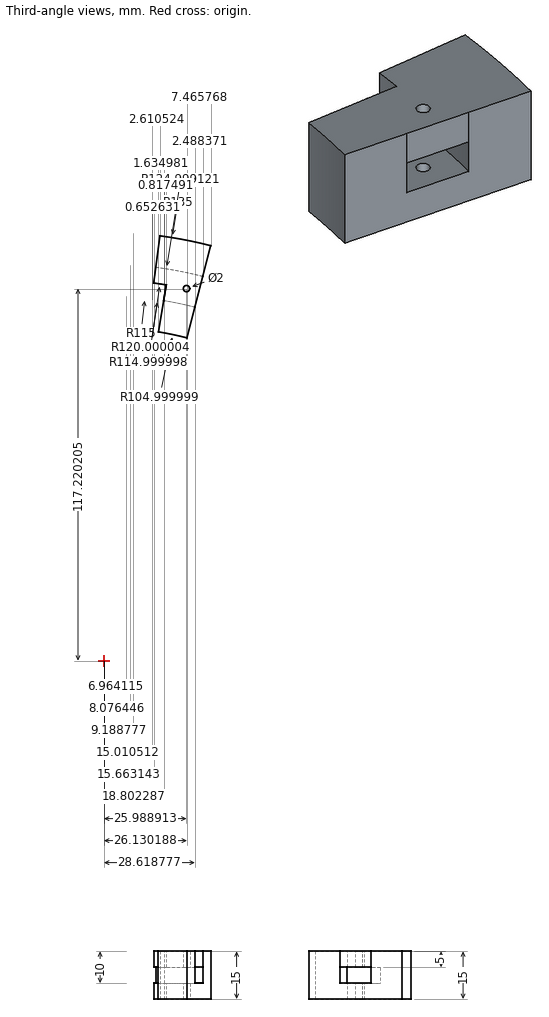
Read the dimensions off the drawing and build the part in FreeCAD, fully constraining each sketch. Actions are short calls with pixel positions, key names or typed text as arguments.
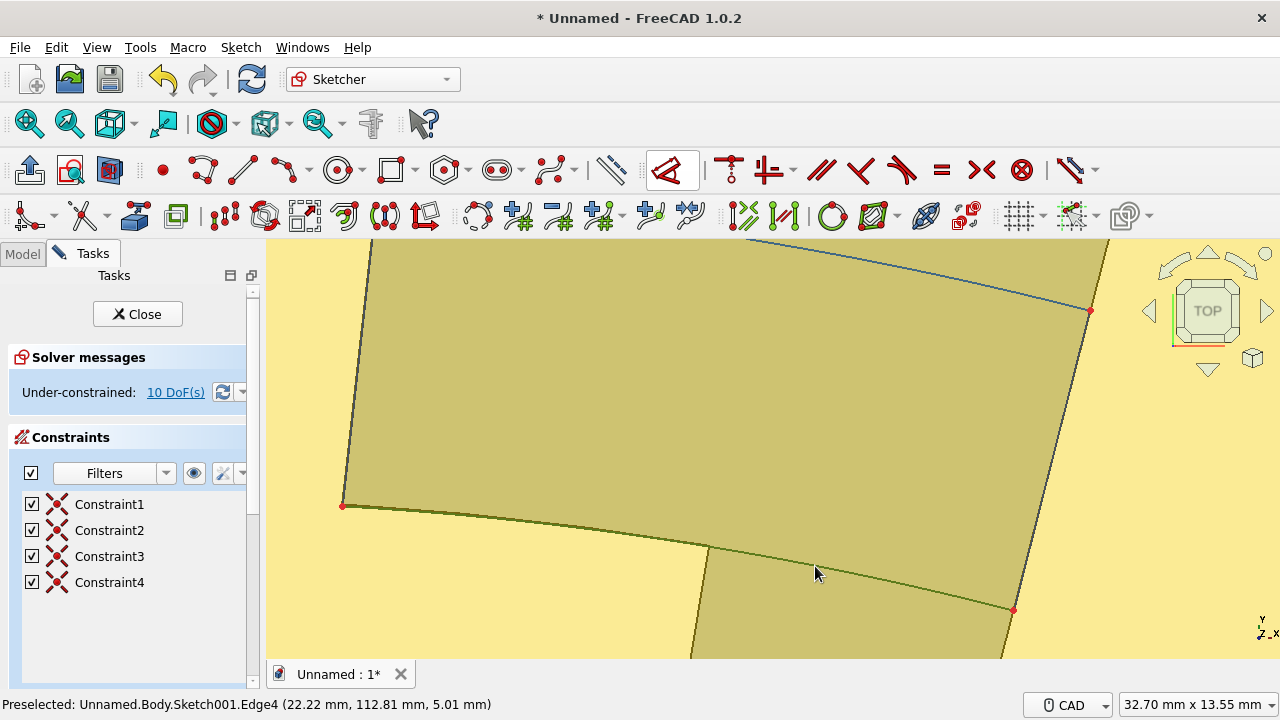
click(730, 170)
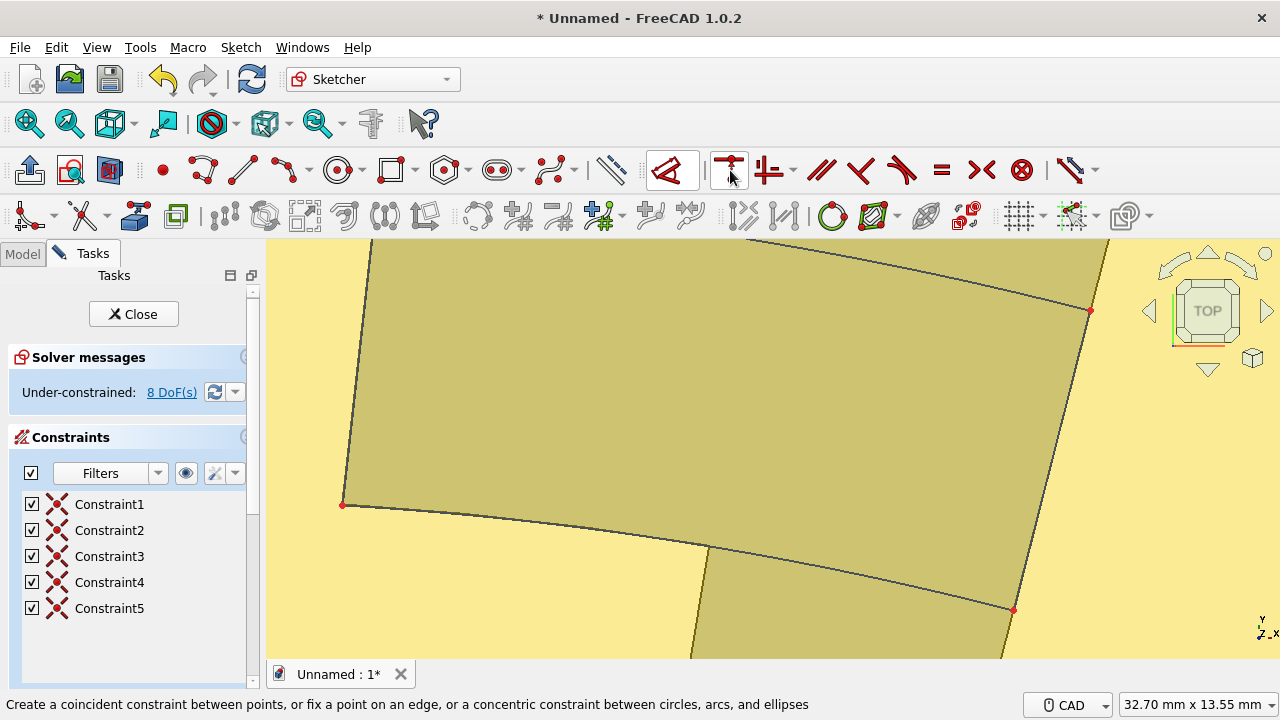
scroll(680, 543, down, 2)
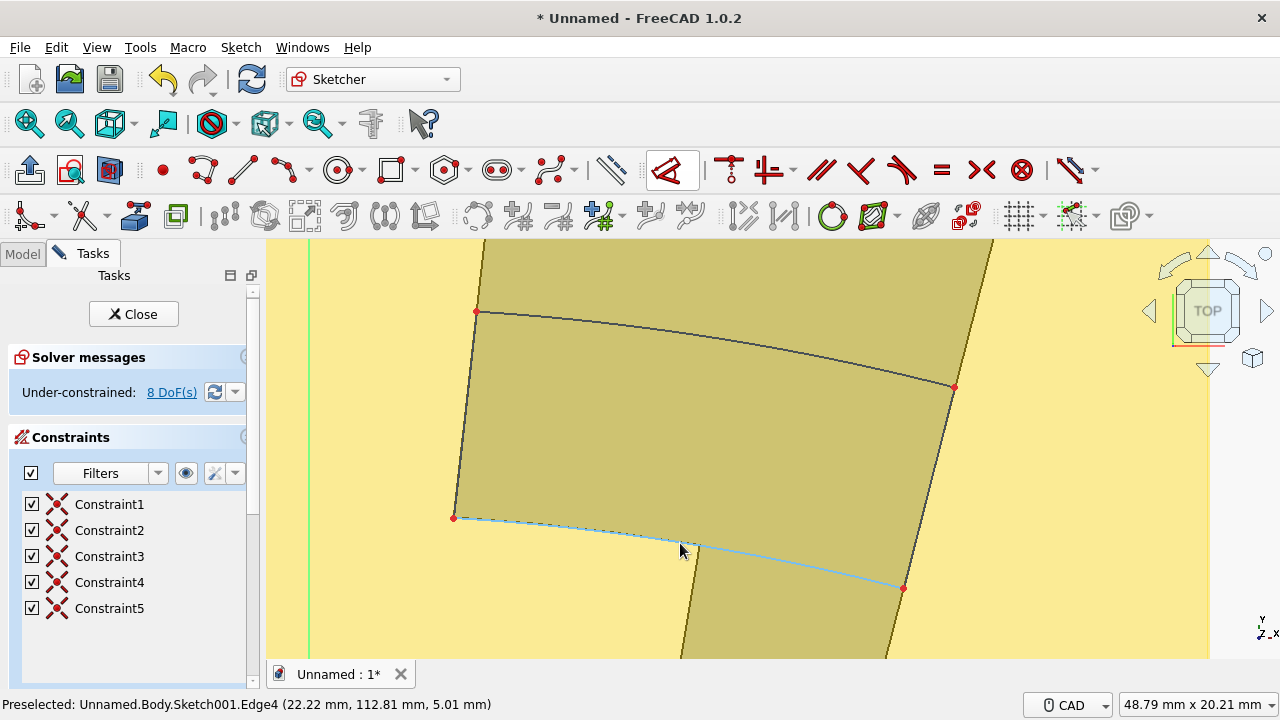
scroll(712, 334, down, 12)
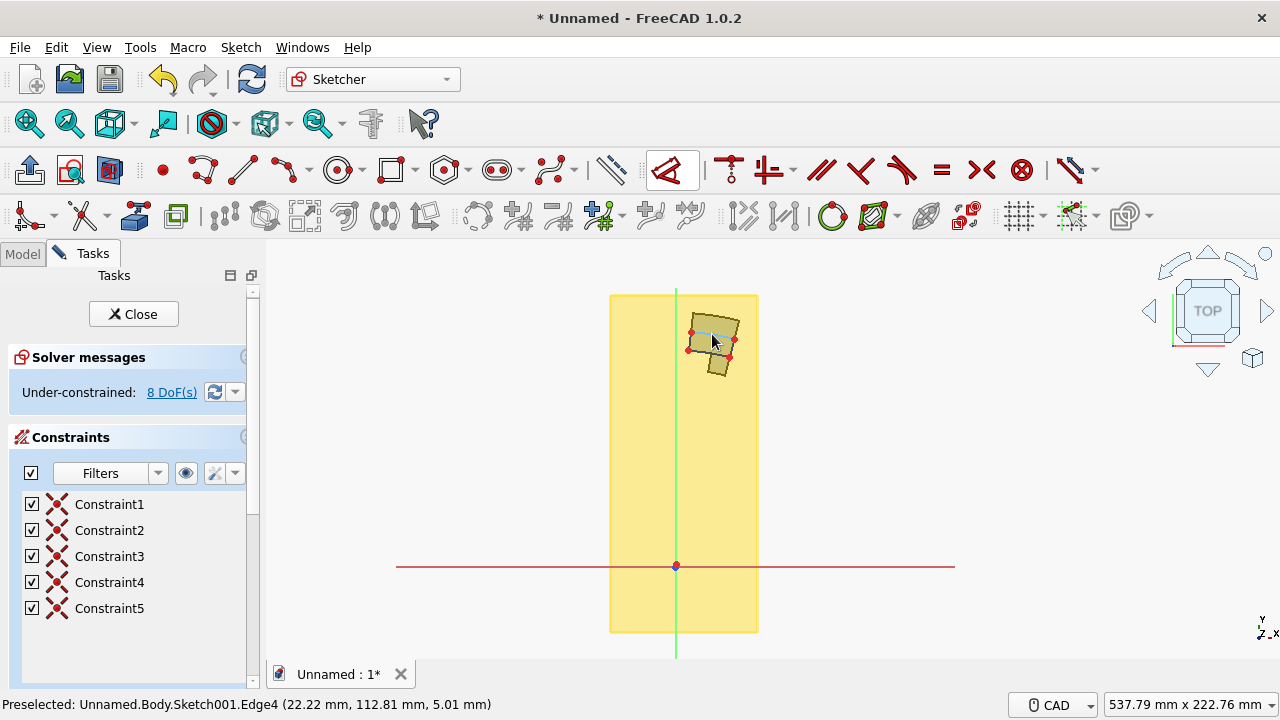
drag(666, 554, 686, 577)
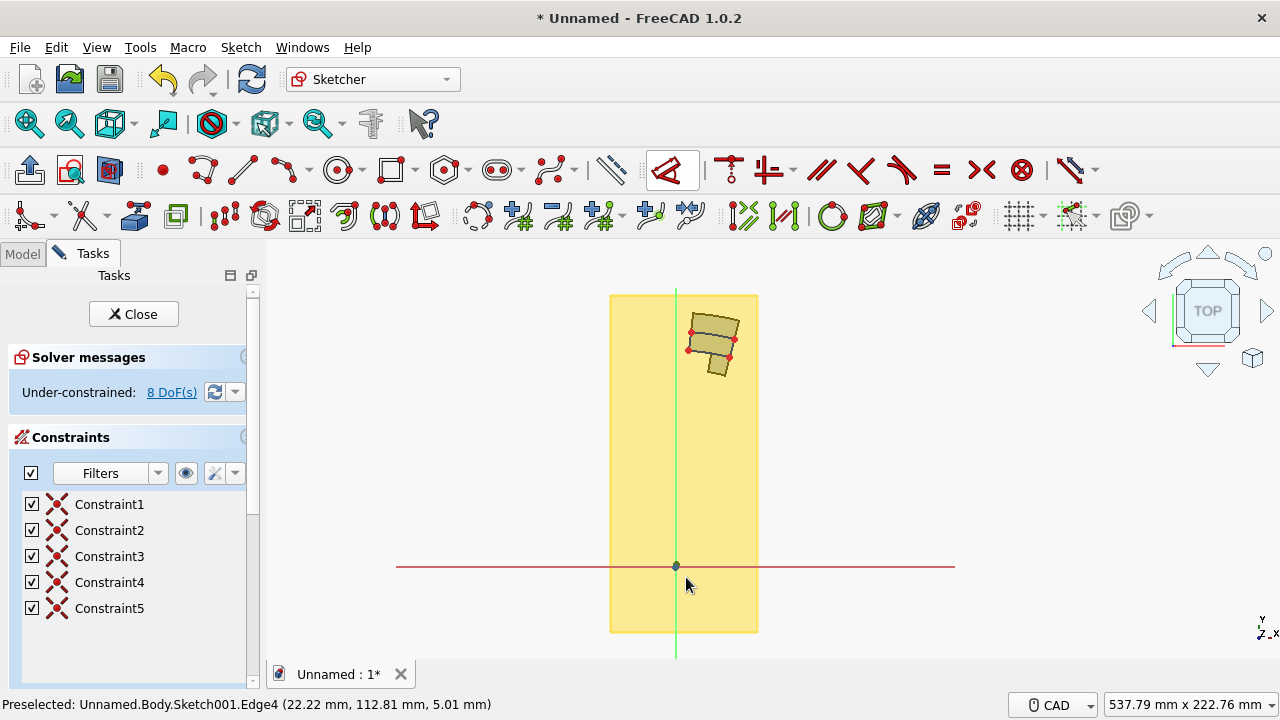
click(730, 170)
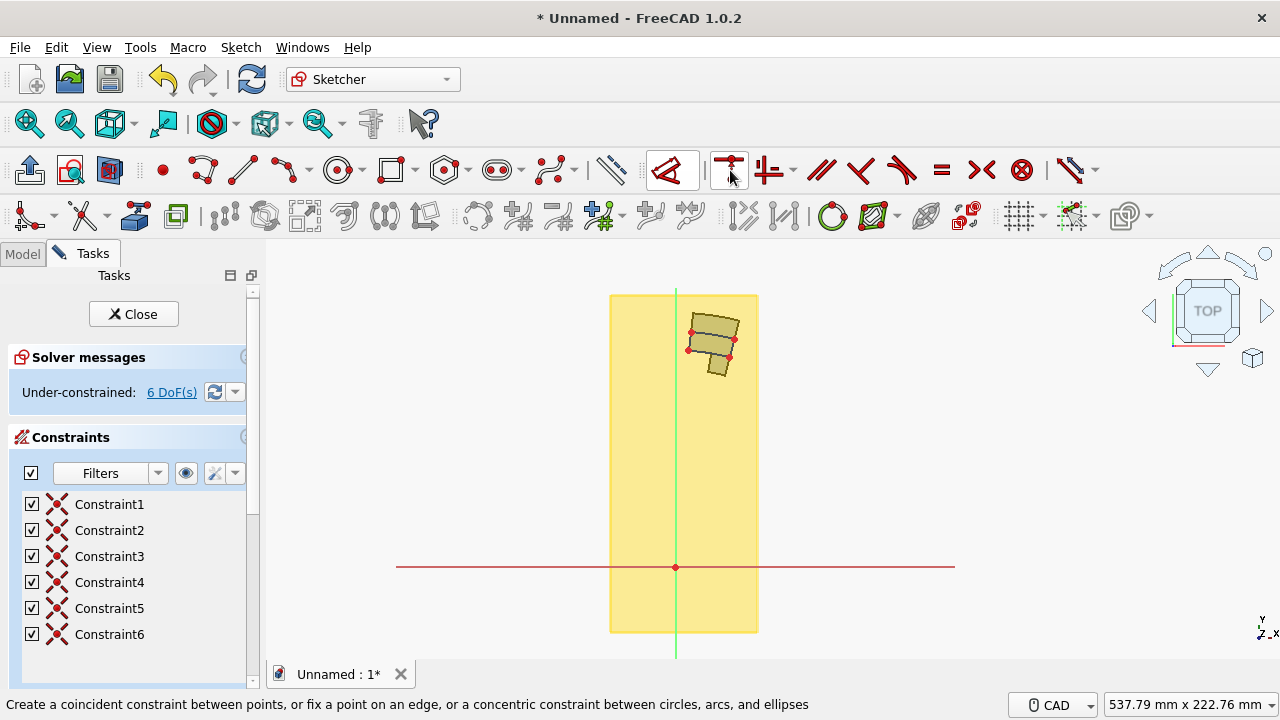
click(722, 336)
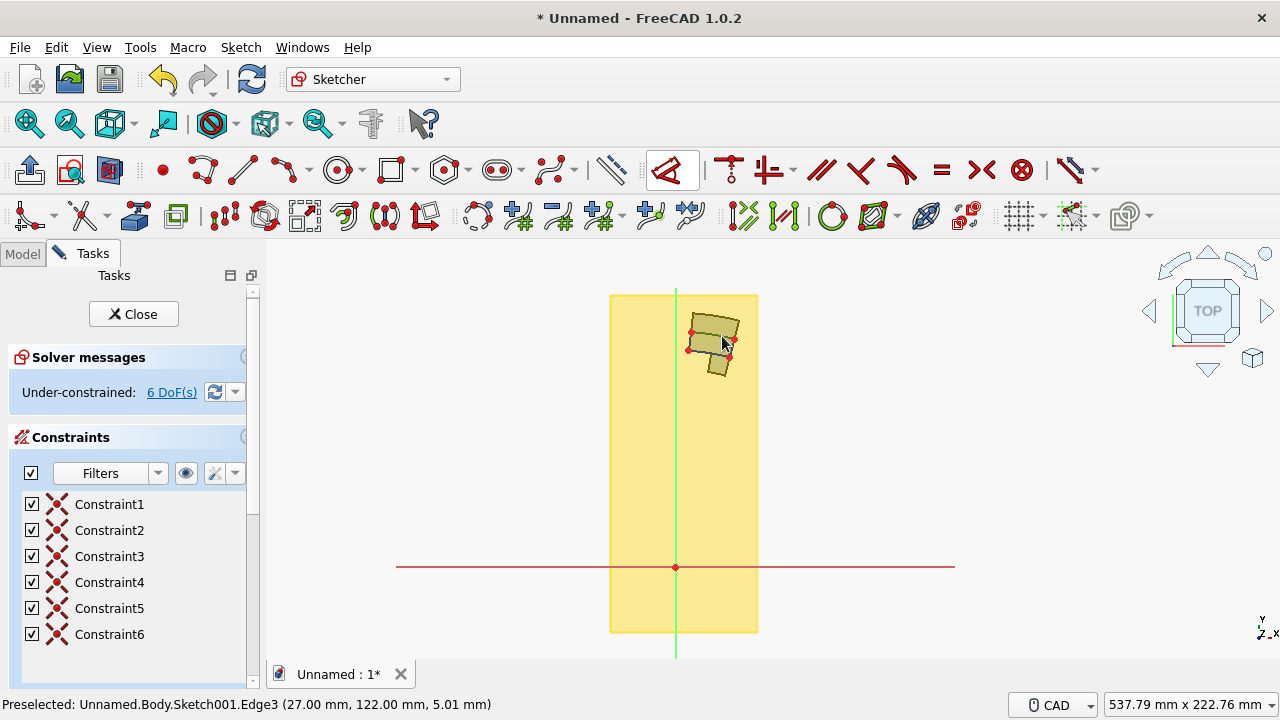
key(k)
key(r)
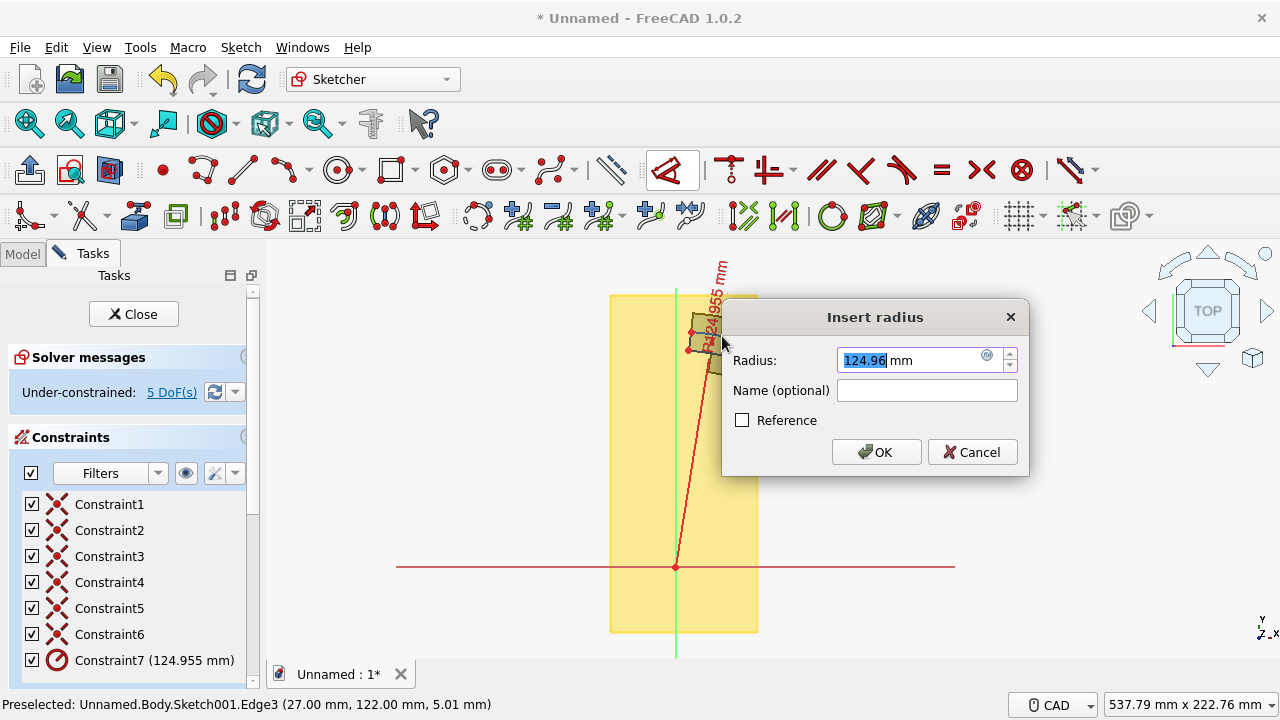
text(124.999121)
key(Return)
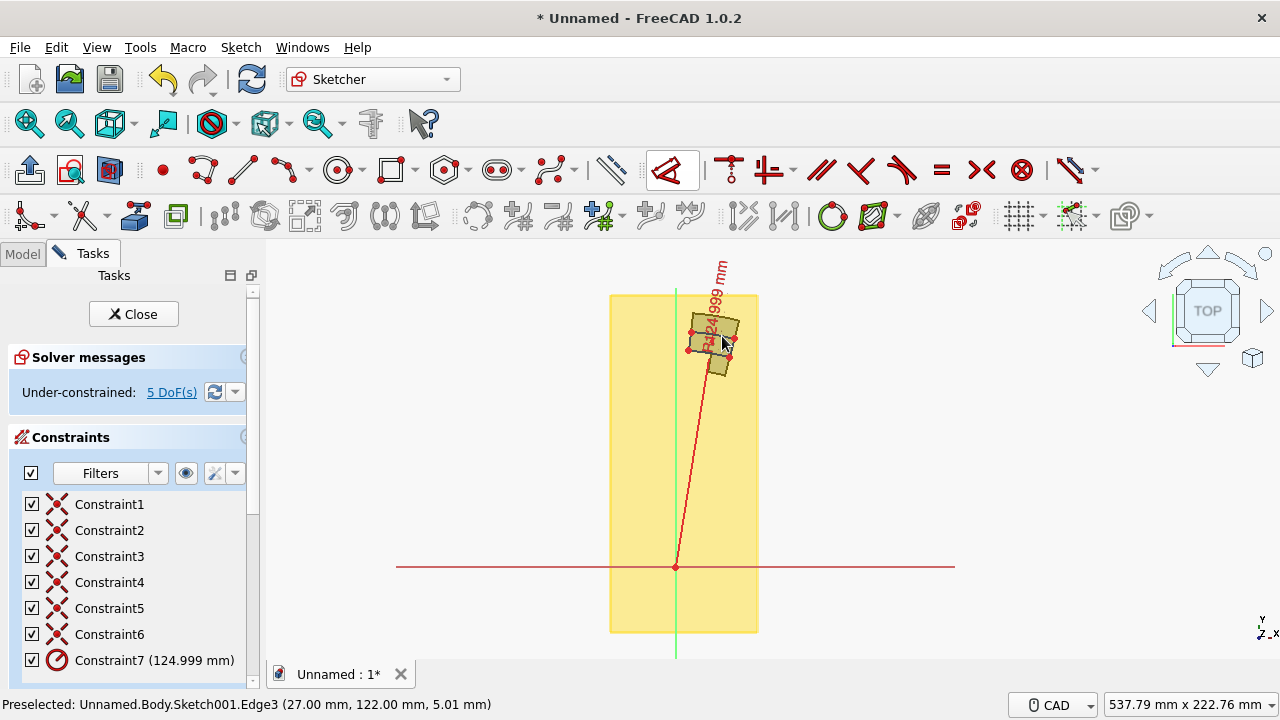
click(718, 355)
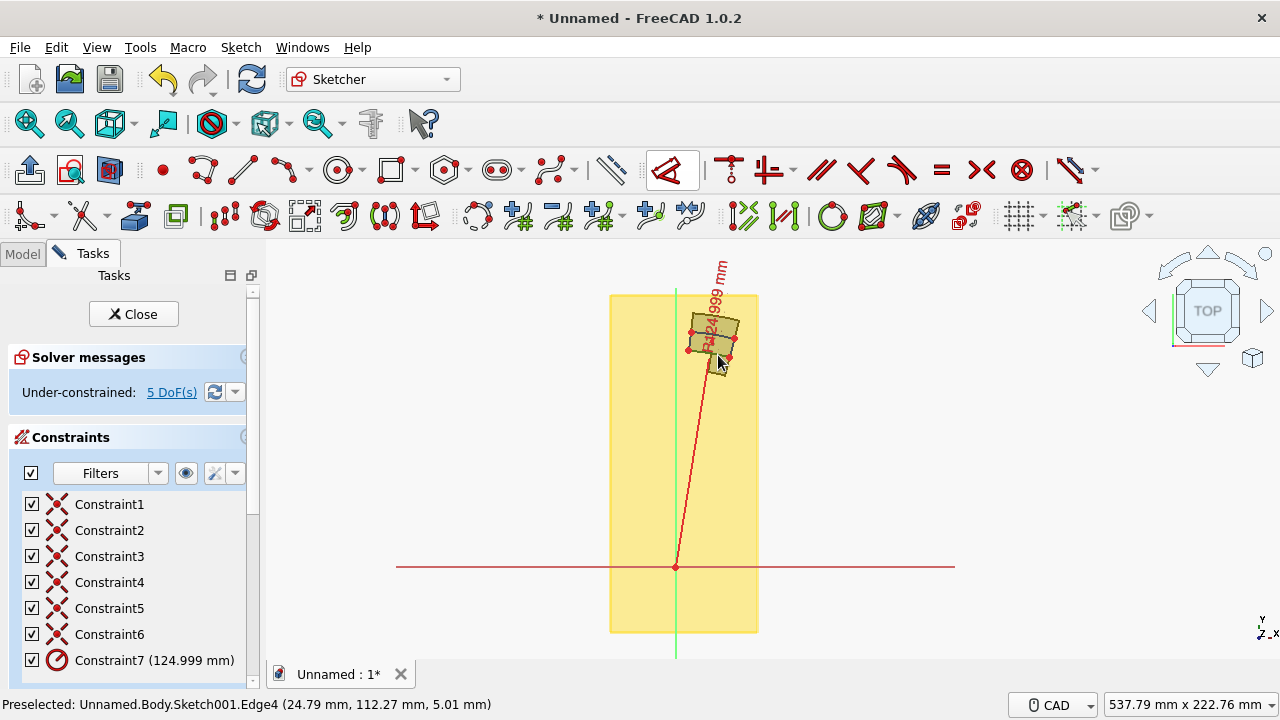
key(k)
key(r)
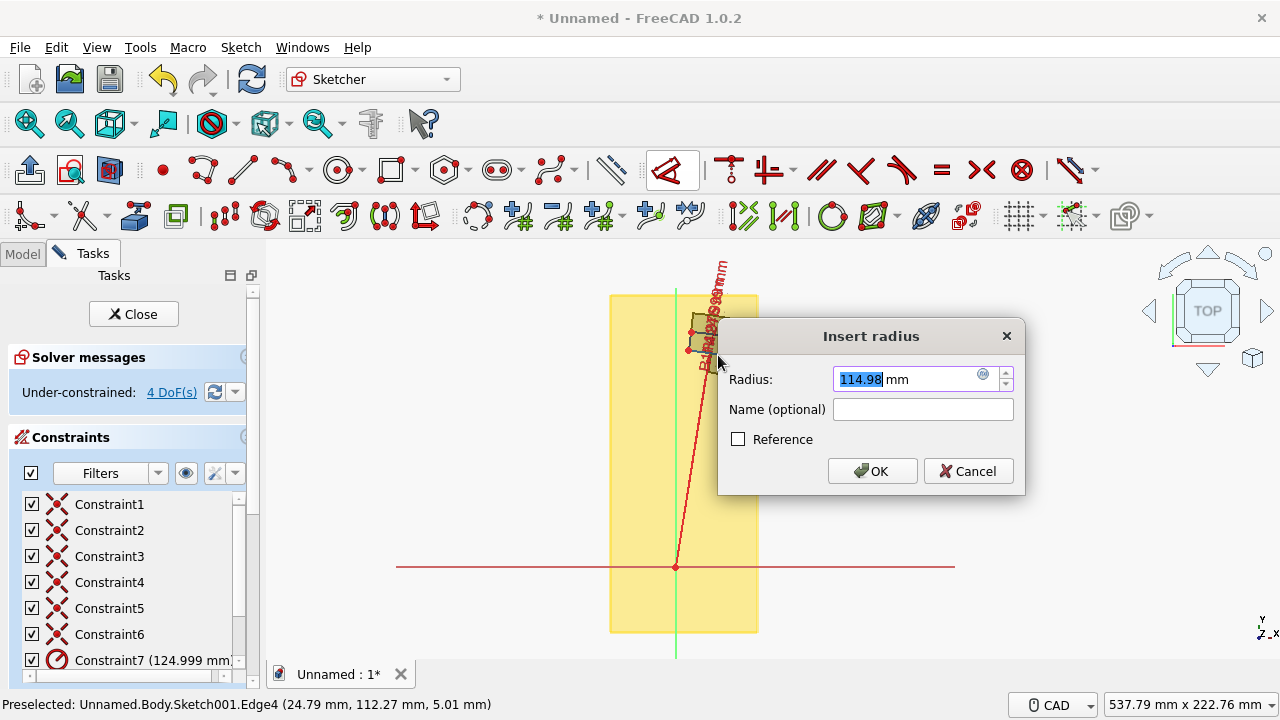
text(115)
key(Return)